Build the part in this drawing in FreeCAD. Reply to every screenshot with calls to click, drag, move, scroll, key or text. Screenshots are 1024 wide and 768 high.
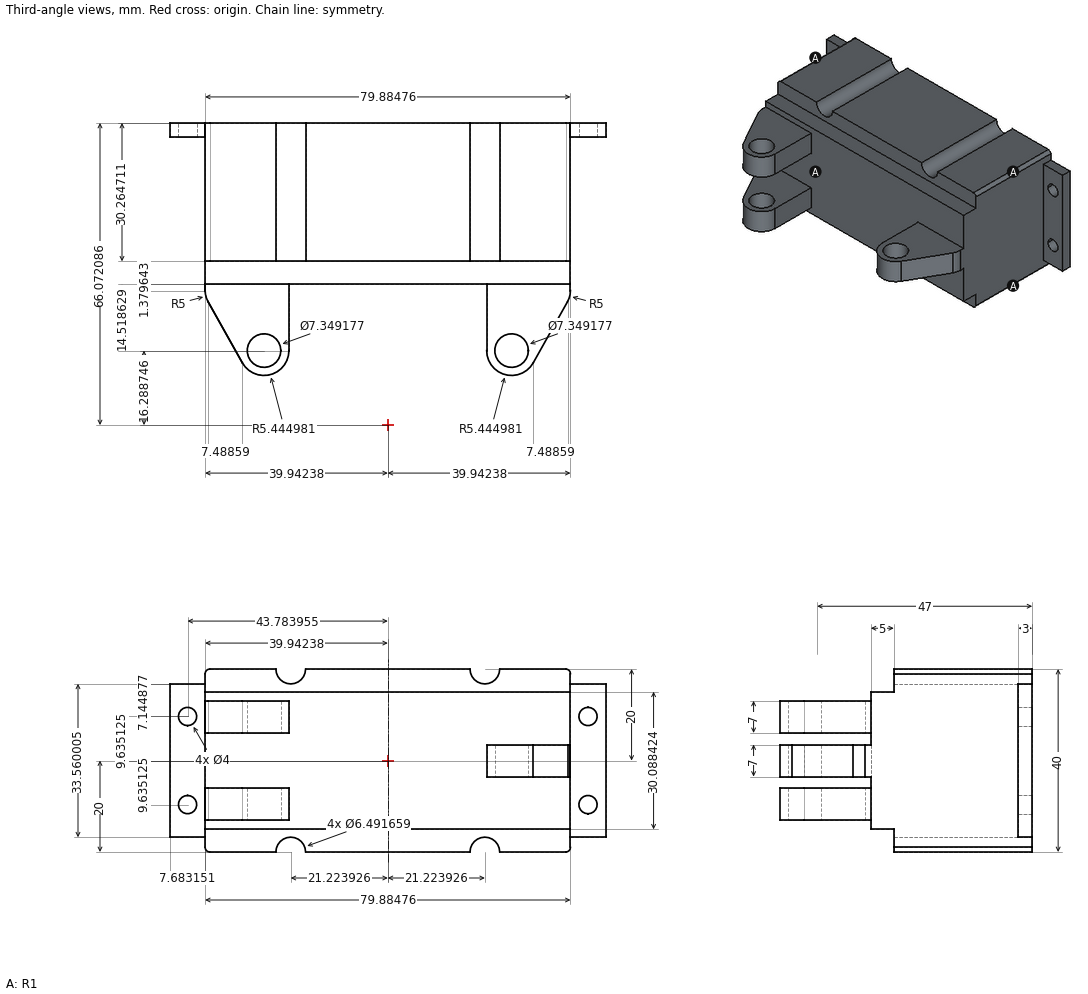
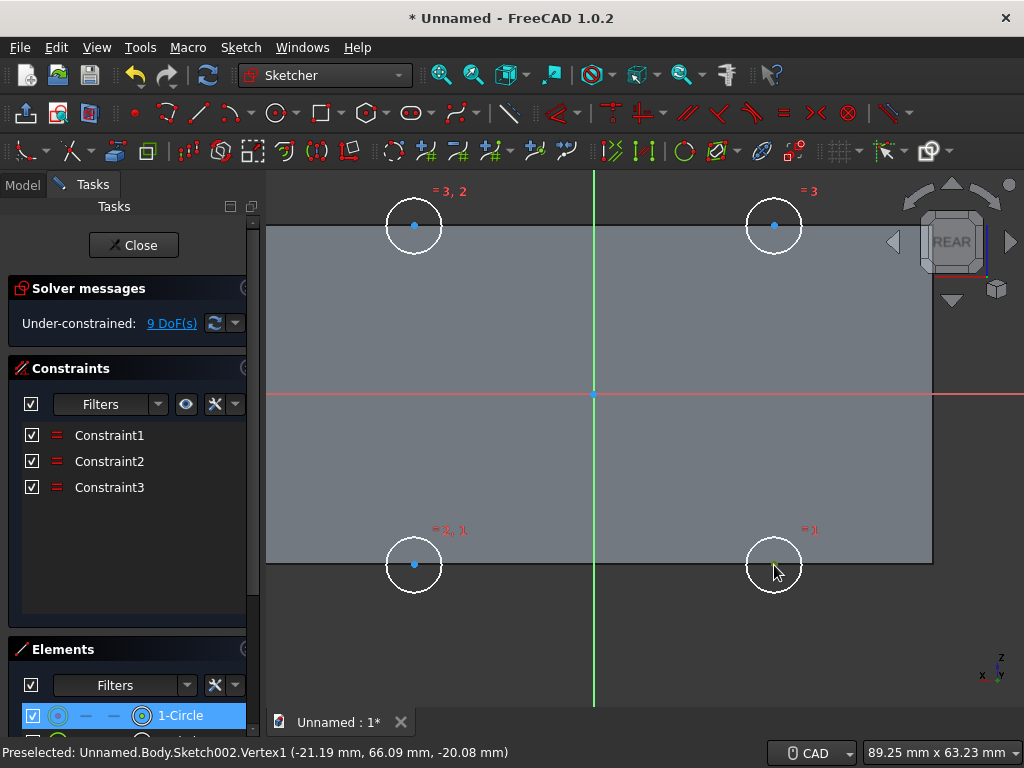
click(414, 565)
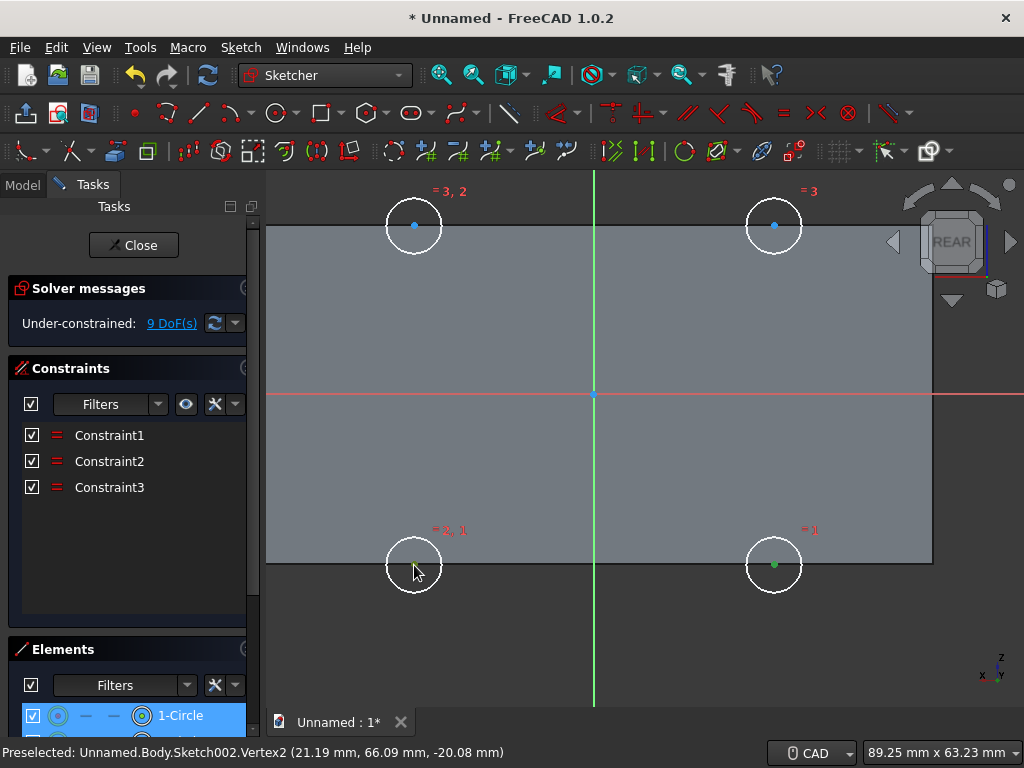
click(666, 114)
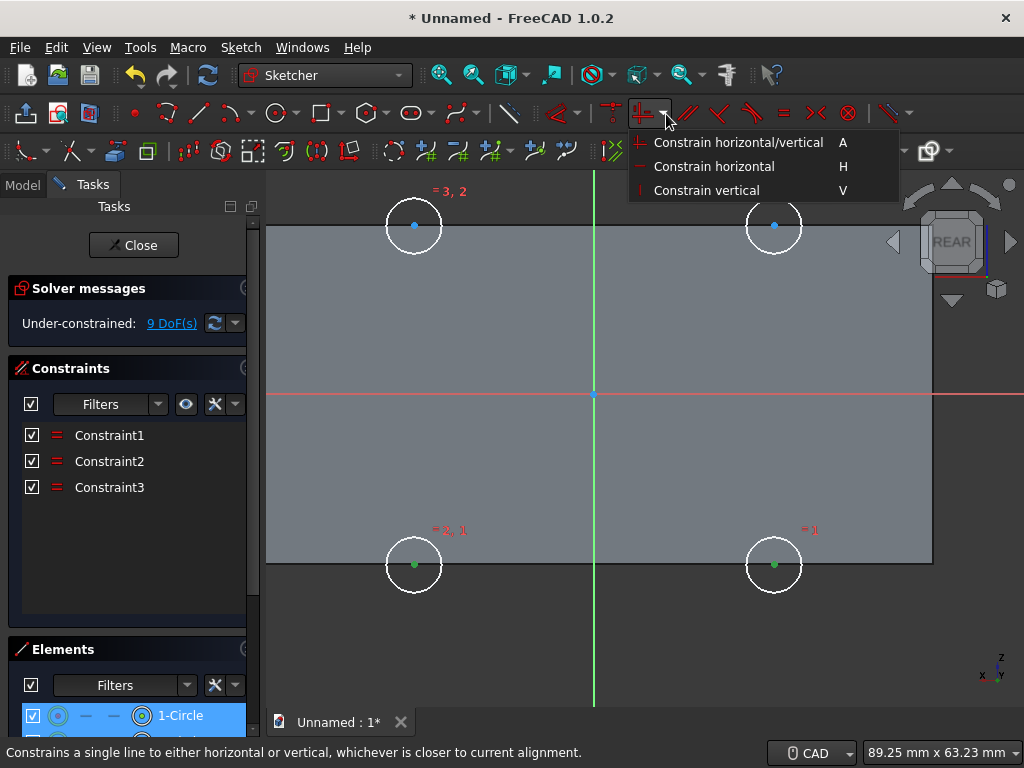
click(764, 166)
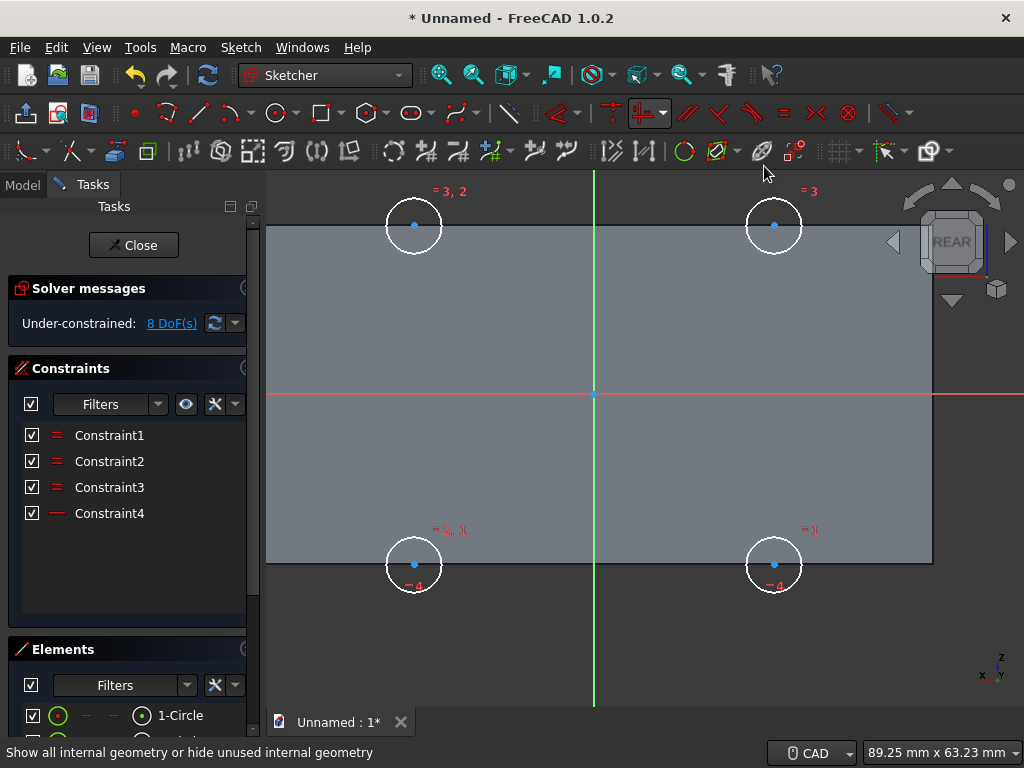
click(414, 565)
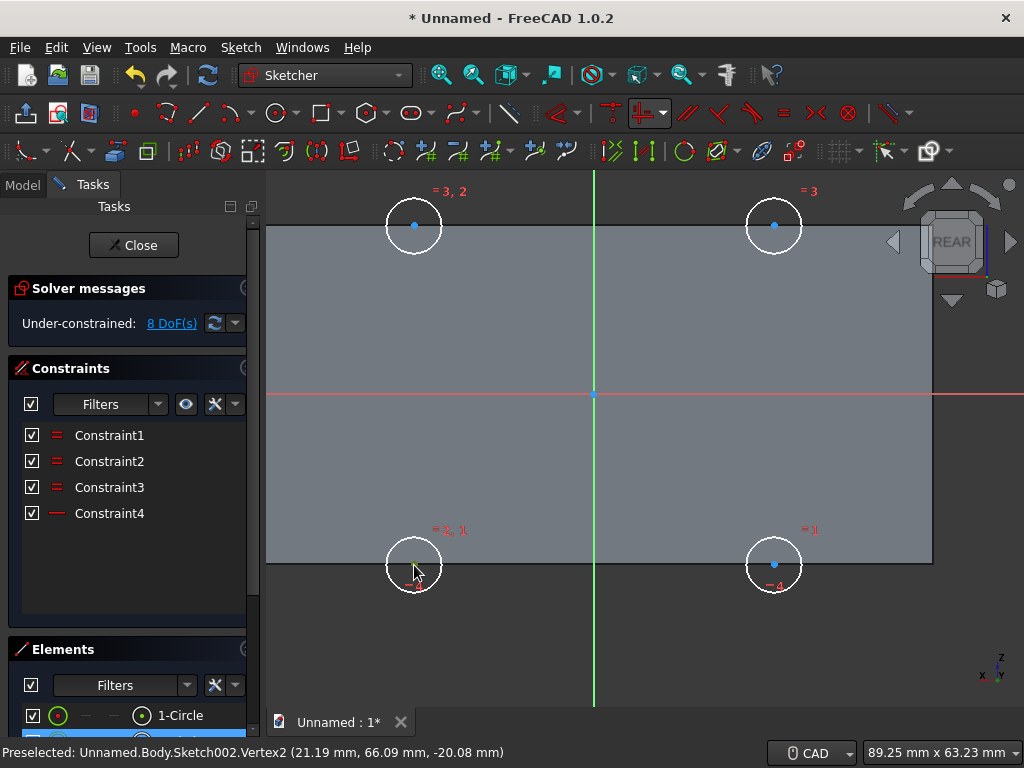
click(414, 226)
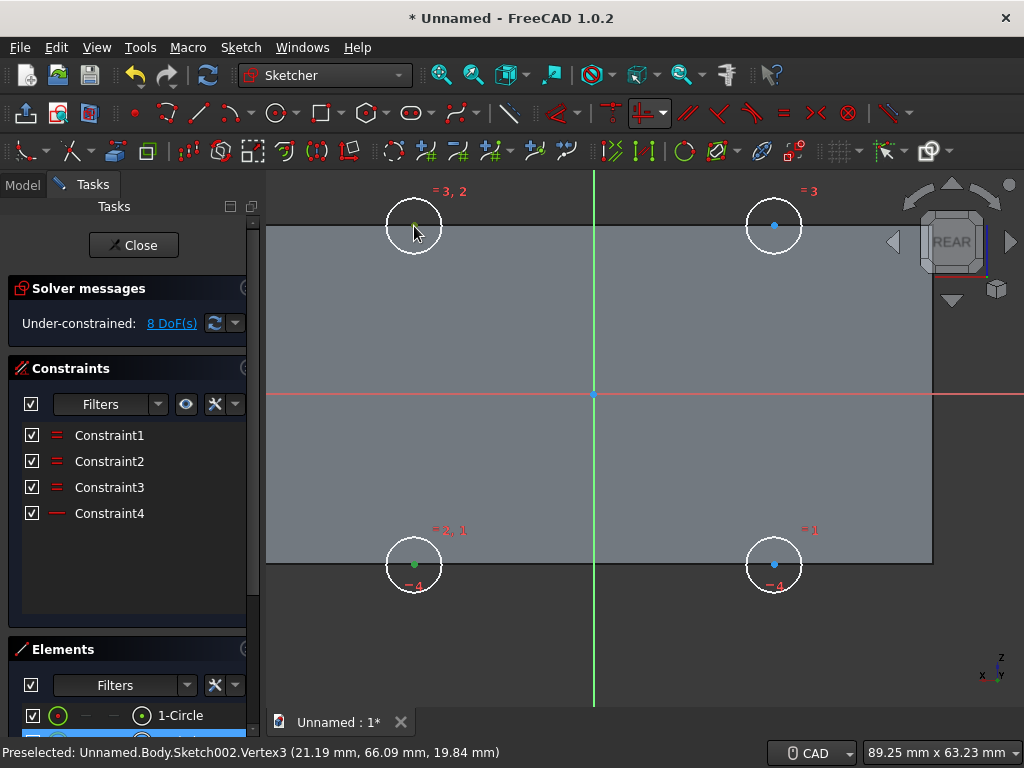
key(v)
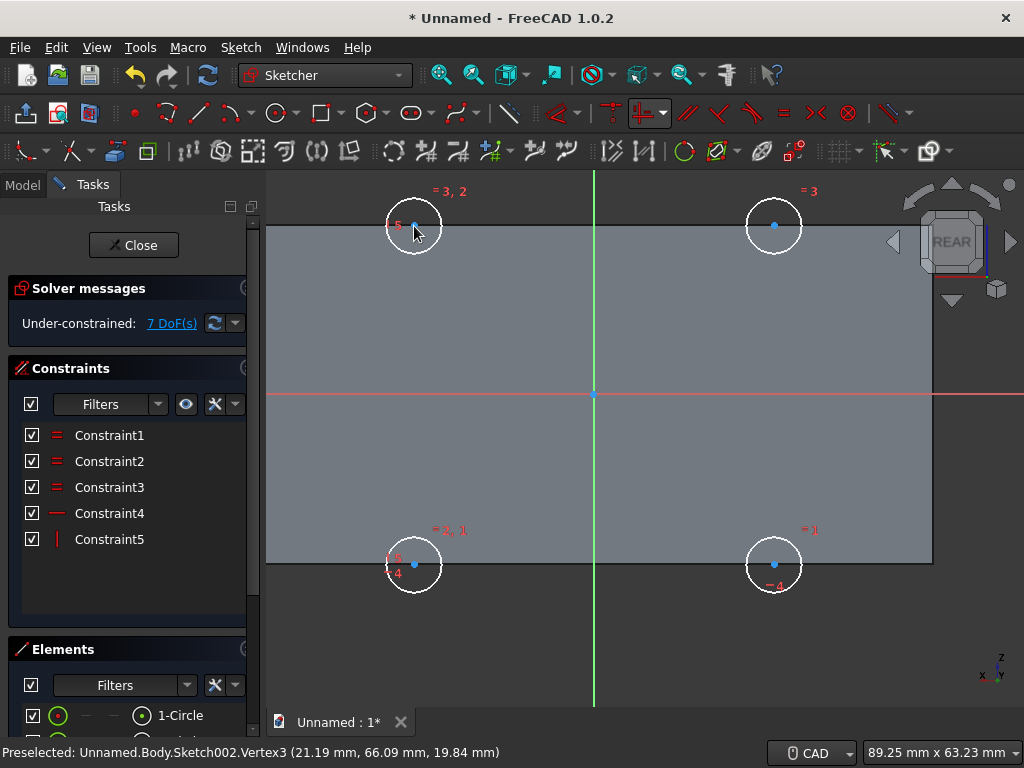
click(774, 565)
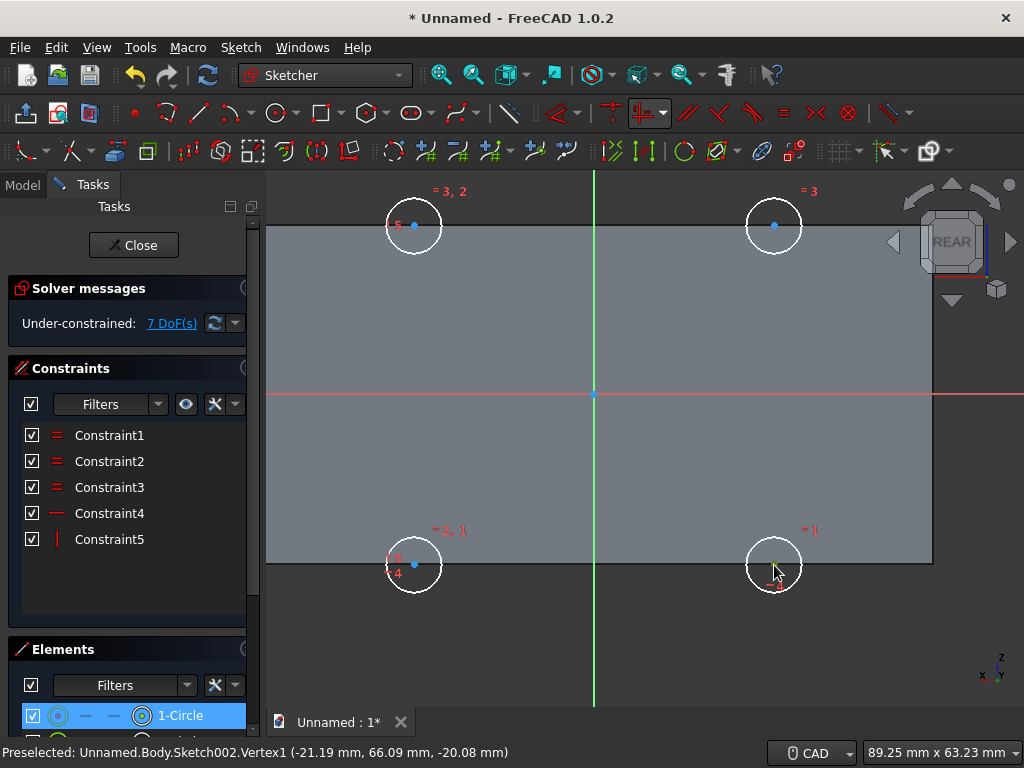
click(774, 226)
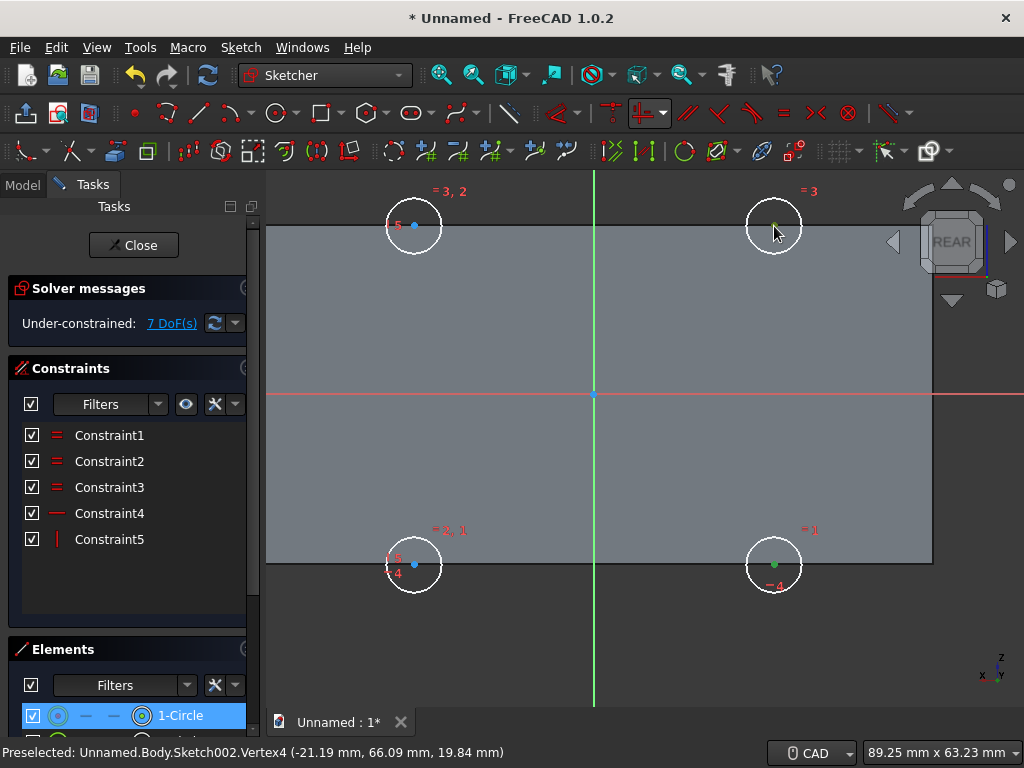
key(v)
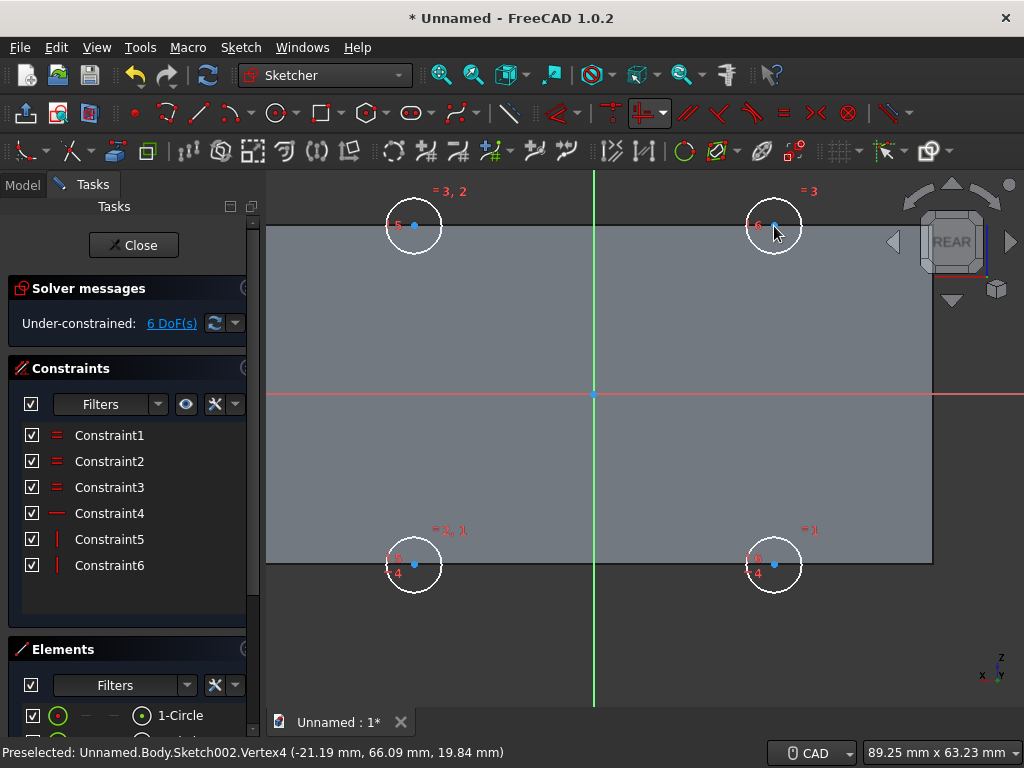
click(414, 226)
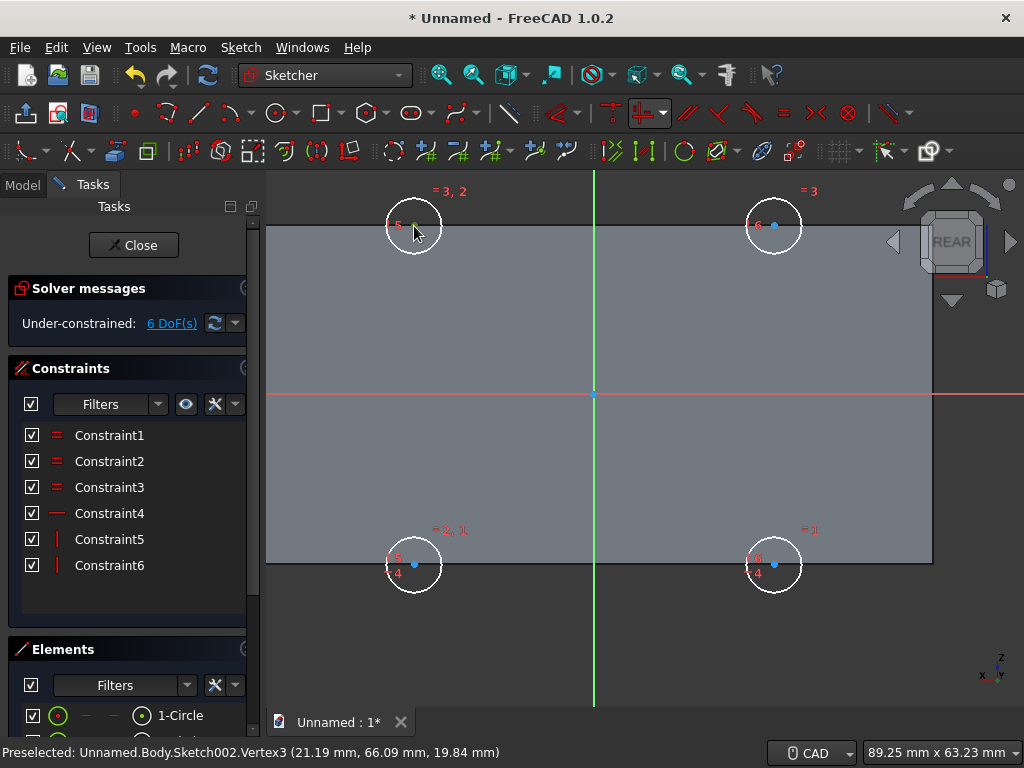
click(774, 226)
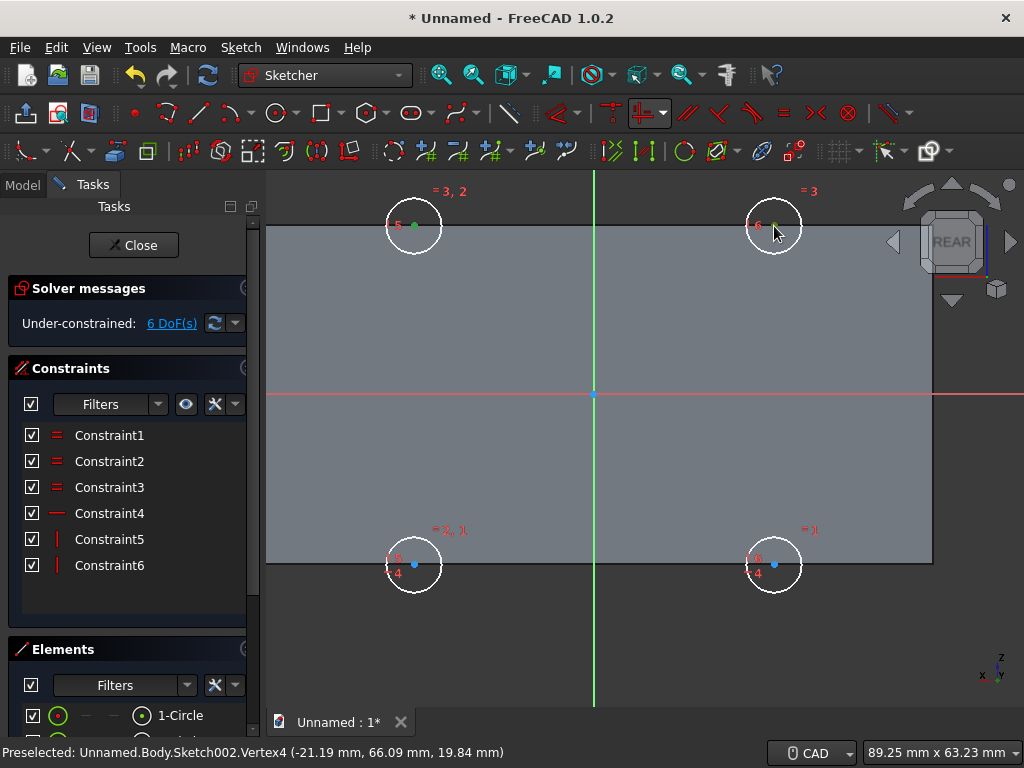
key(h)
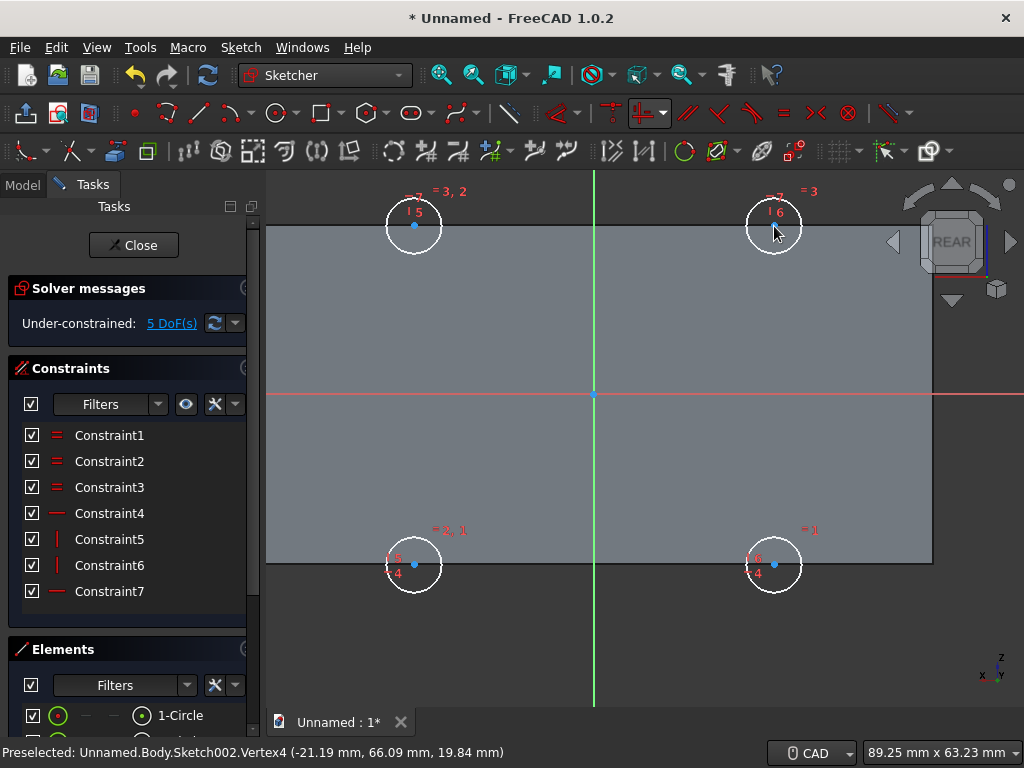
click(556, 114)